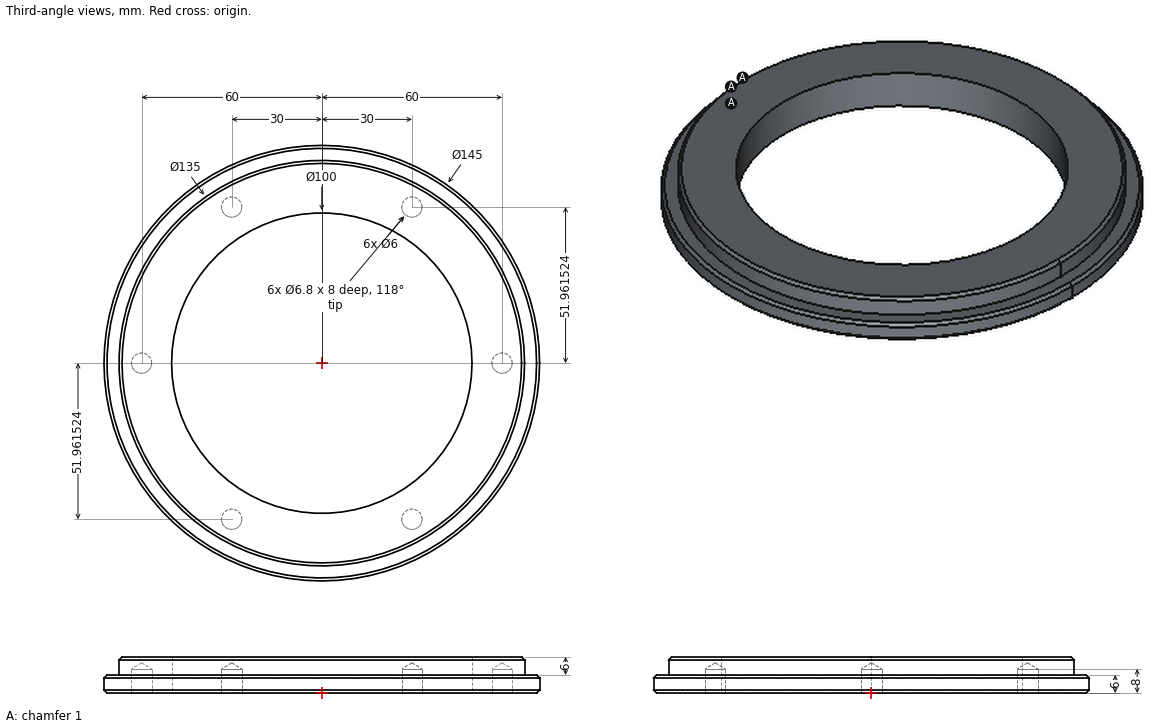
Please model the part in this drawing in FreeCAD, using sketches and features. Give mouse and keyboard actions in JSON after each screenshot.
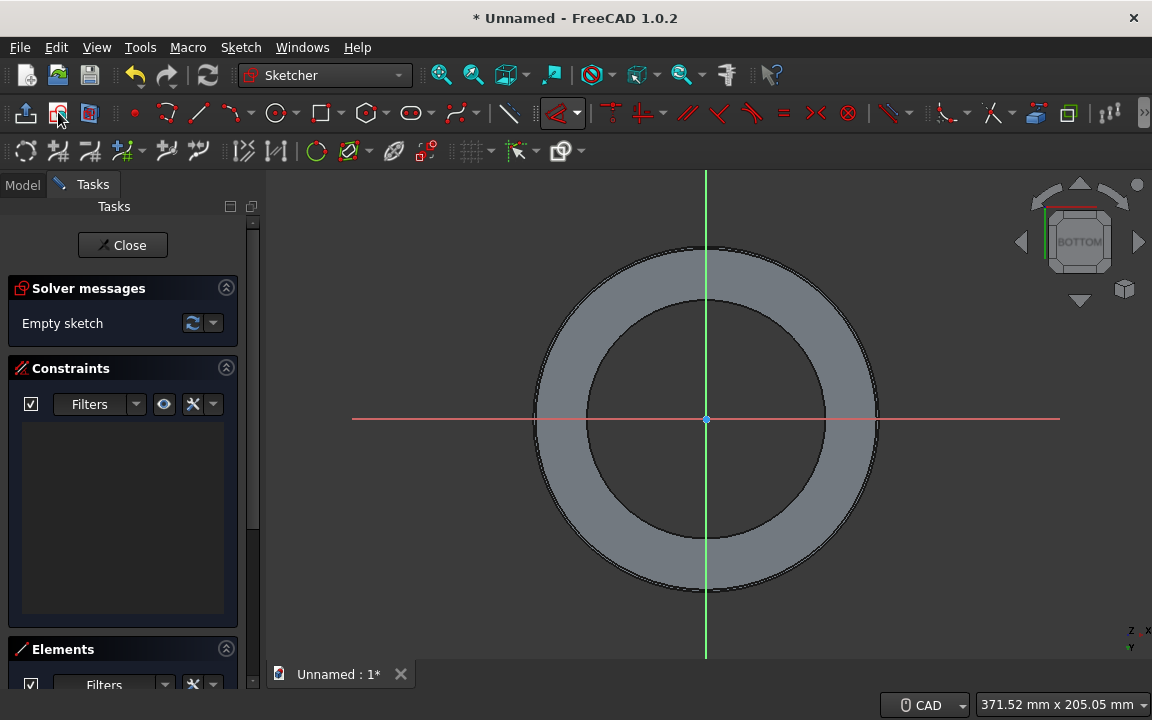
{"action": "left_click", "coordinate": [276, 114]}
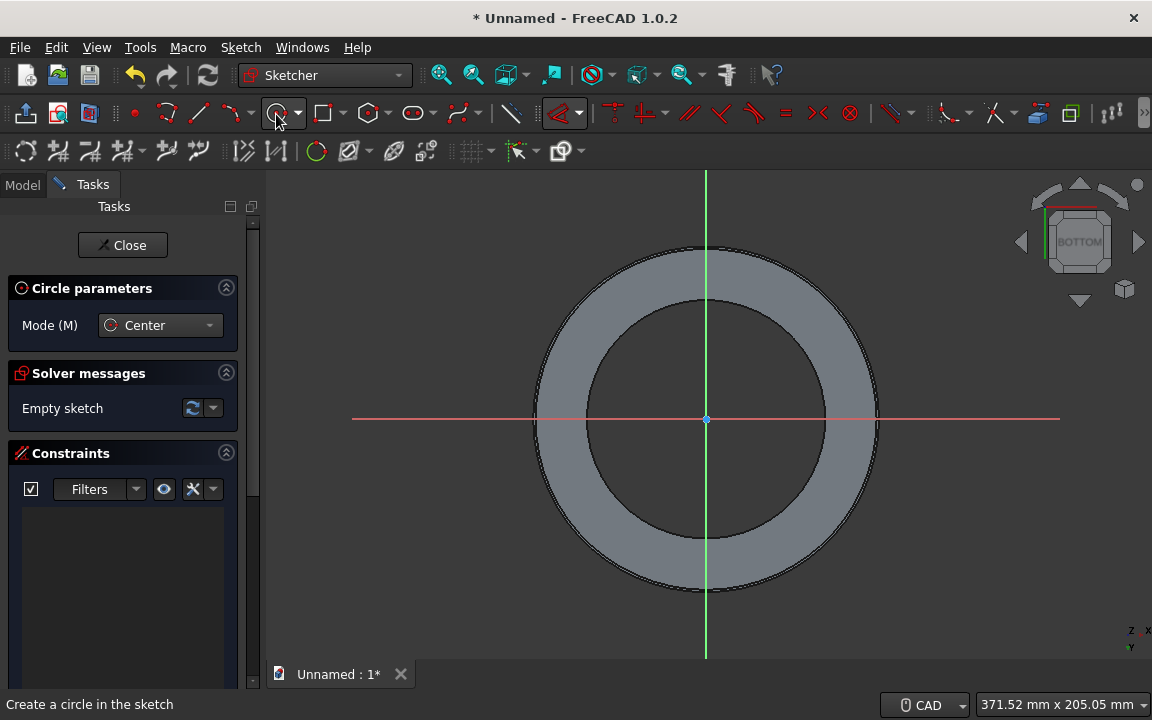
{"action": "scroll", "coordinate": [778, 543], "scroll_direction": "up", "scroll_amount": 6}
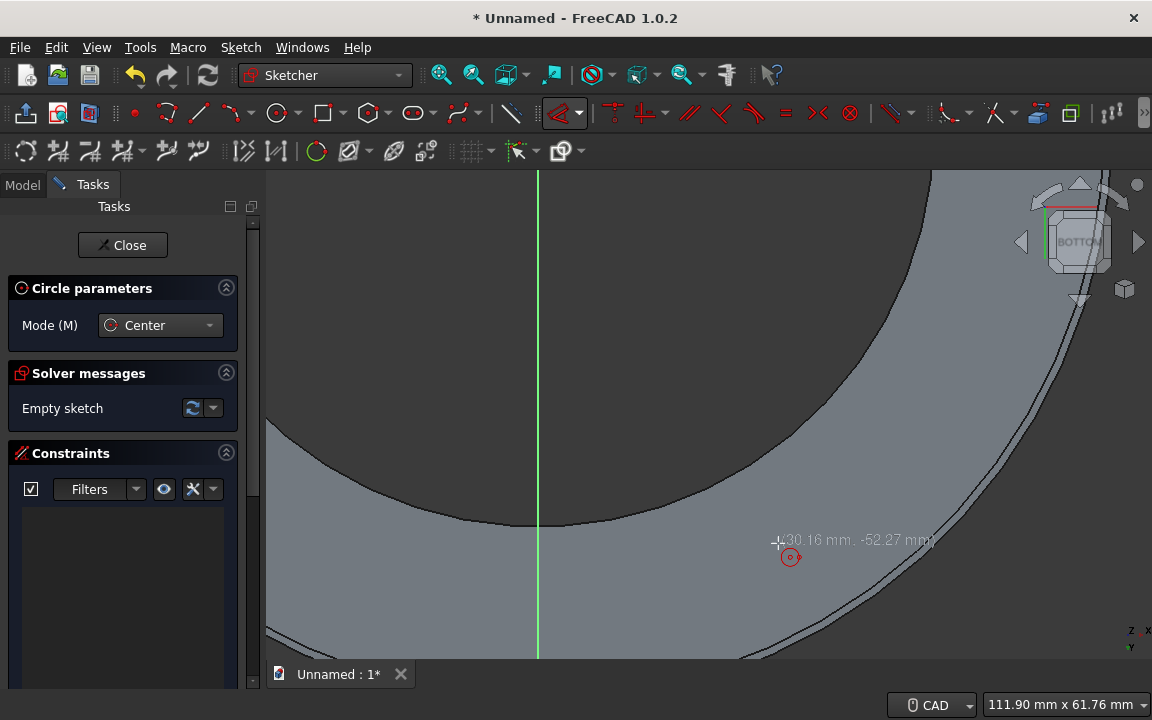
{"action": "left_click", "coordinate": [775, 542]}
{"action": "mouse_move", "coordinate": [792, 525]}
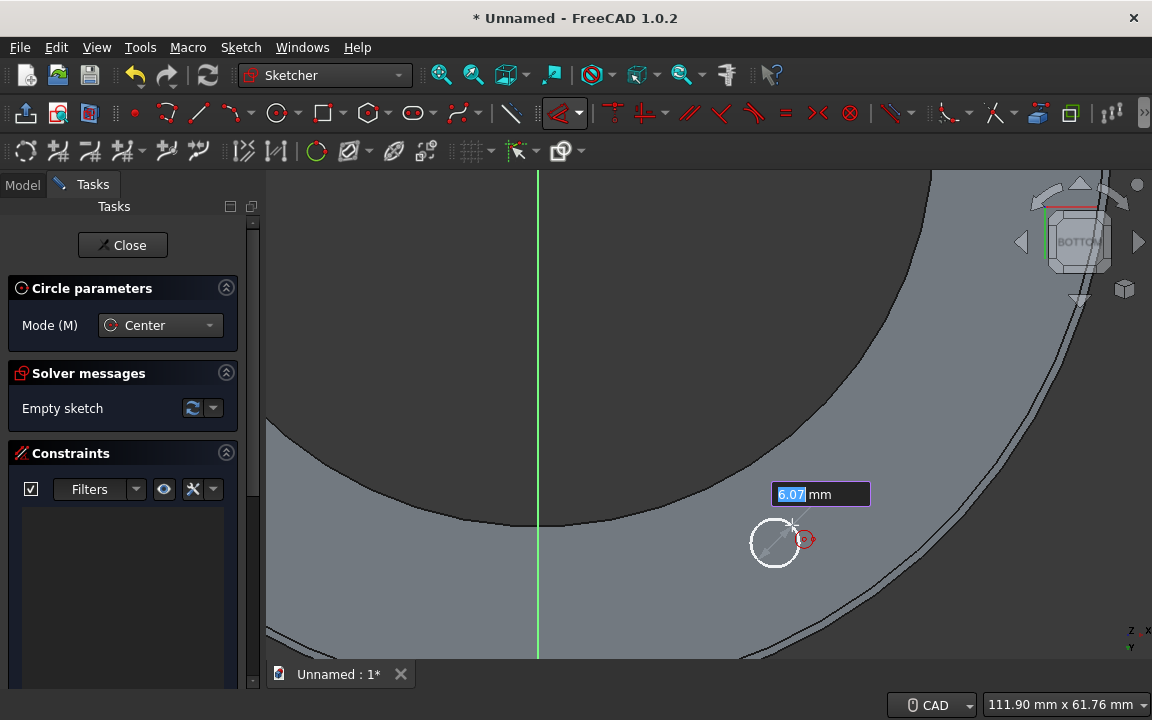
{"action": "type", "text": "6"}
{"action": "key", "text": "Return"}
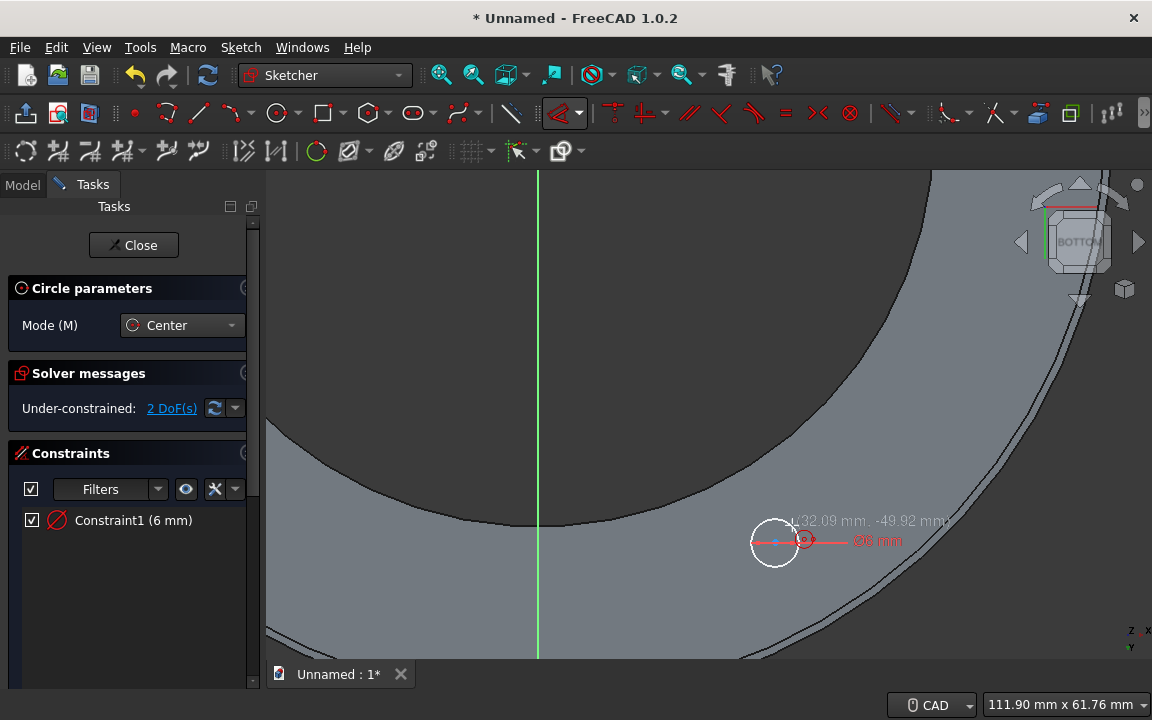
{"action": "scroll", "coordinate": [700, 580], "scroll_direction": "down", "scroll_amount": 5}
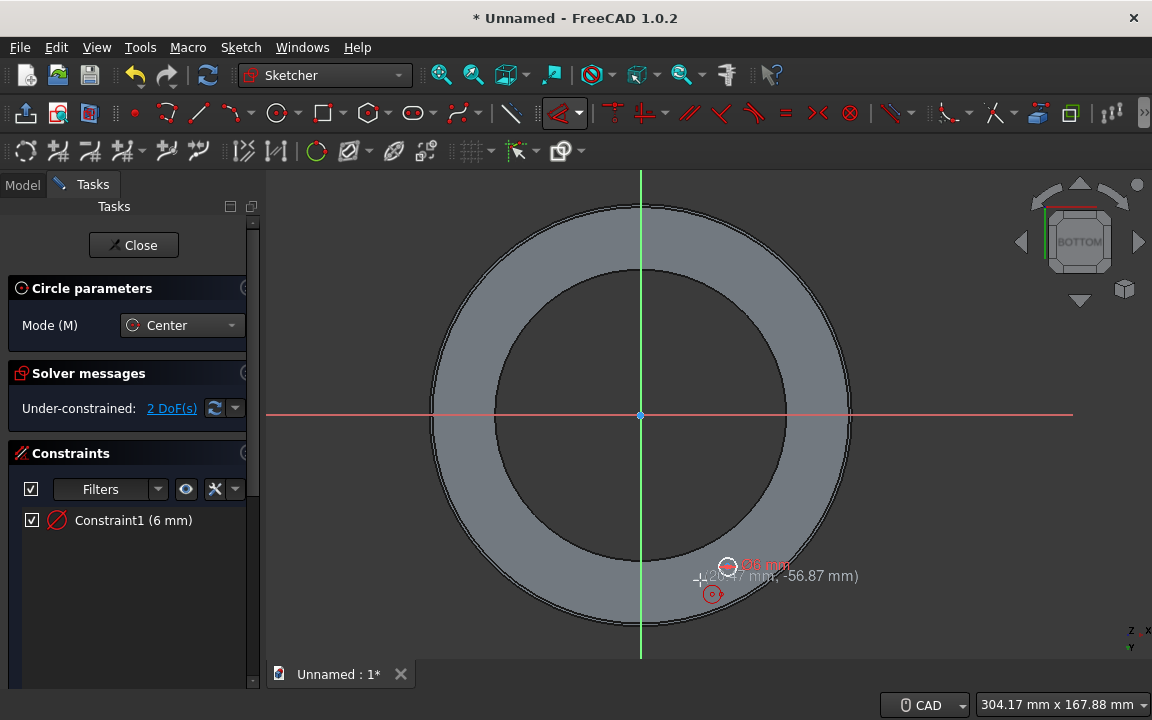
{"action": "scroll", "coordinate": [815, 415], "scroll_direction": "up", "scroll_amount": 5}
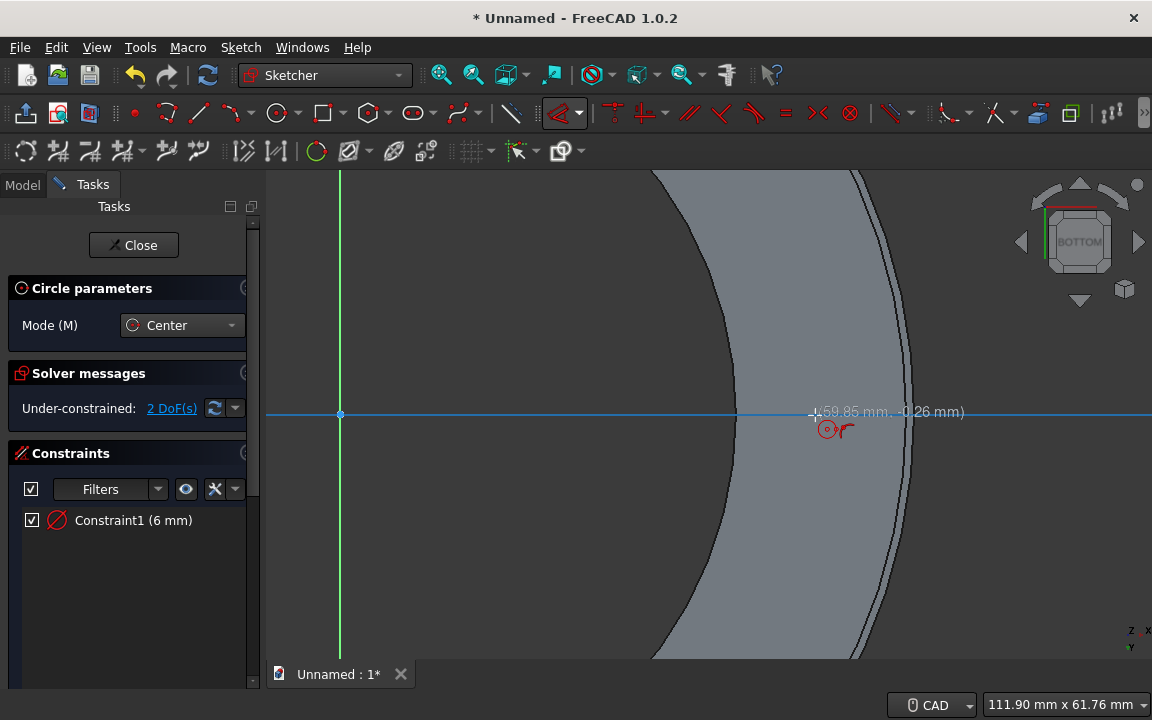
{"action": "left_click", "coordinate": [815, 415]}
{"action": "mouse_move", "coordinate": [832, 398]}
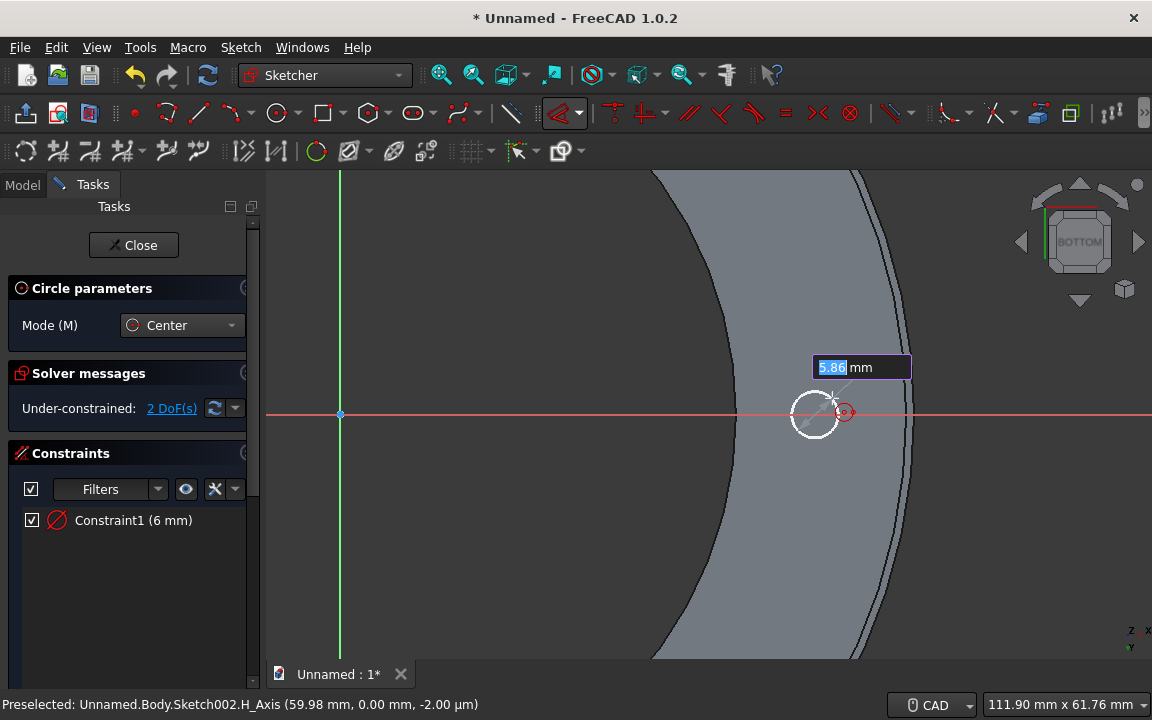
{"action": "type", "text": "6"}
{"action": "key", "text": "Return"}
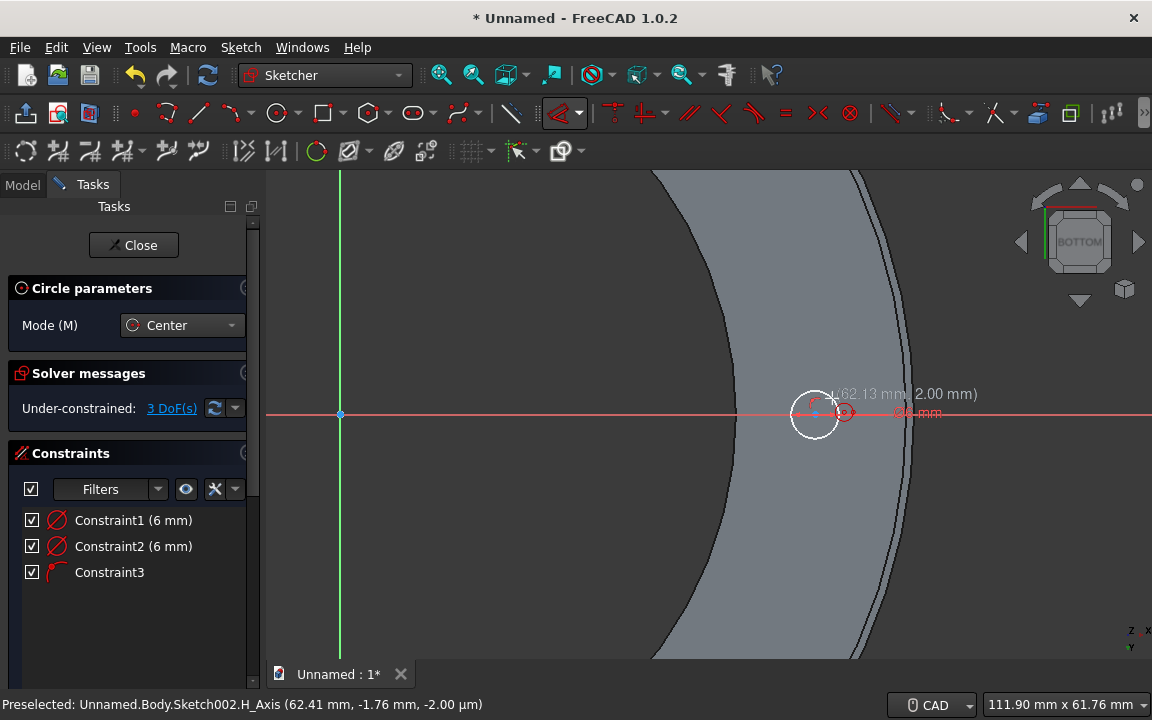
{"action": "scroll", "coordinate": [815, 414], "scroll_direction": "down", "scroll_amount": 5}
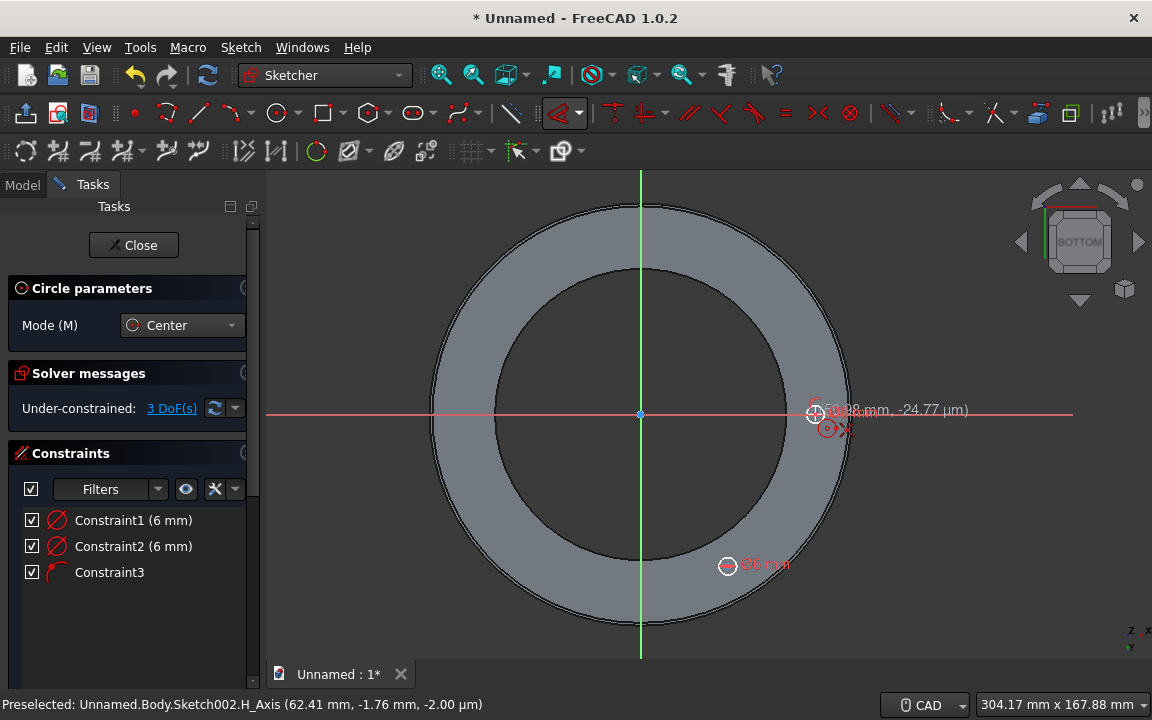
{"action": "scroll", "coordinate": [553, 566], "scroll_direction": "up", "scroll_amount": 5}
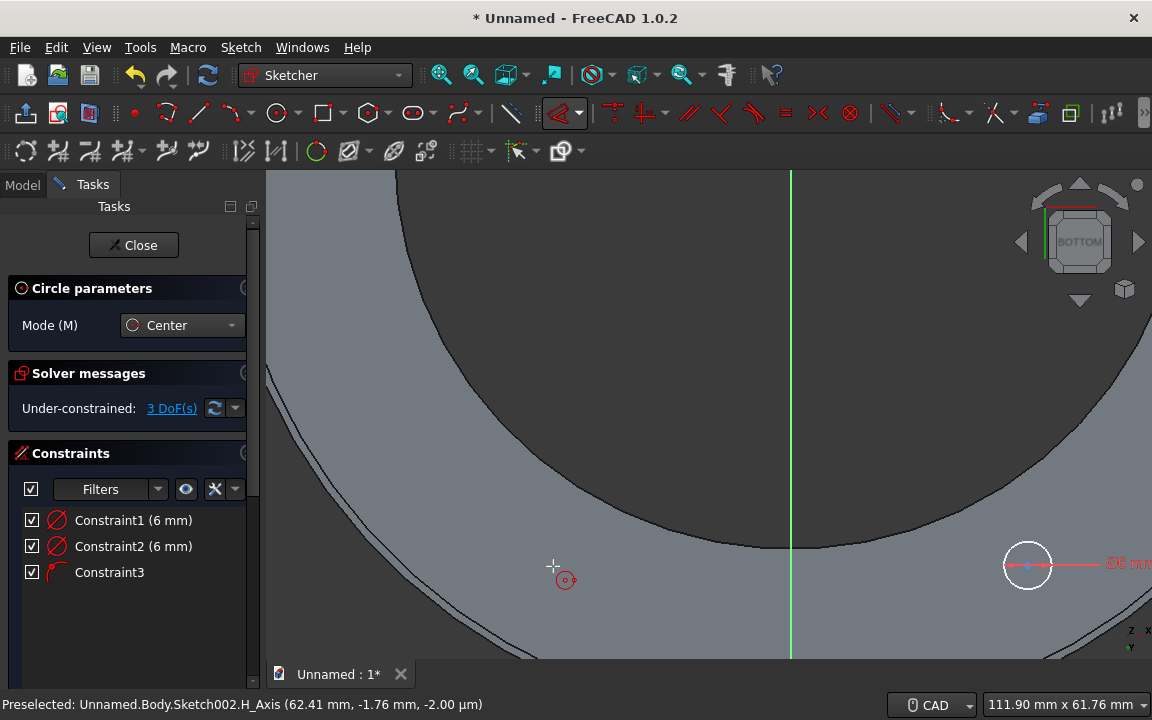
{"action": "left_click", "coordinate": [553, 565]}
{"action": "mouse_move", "coordinate": [570, 548]}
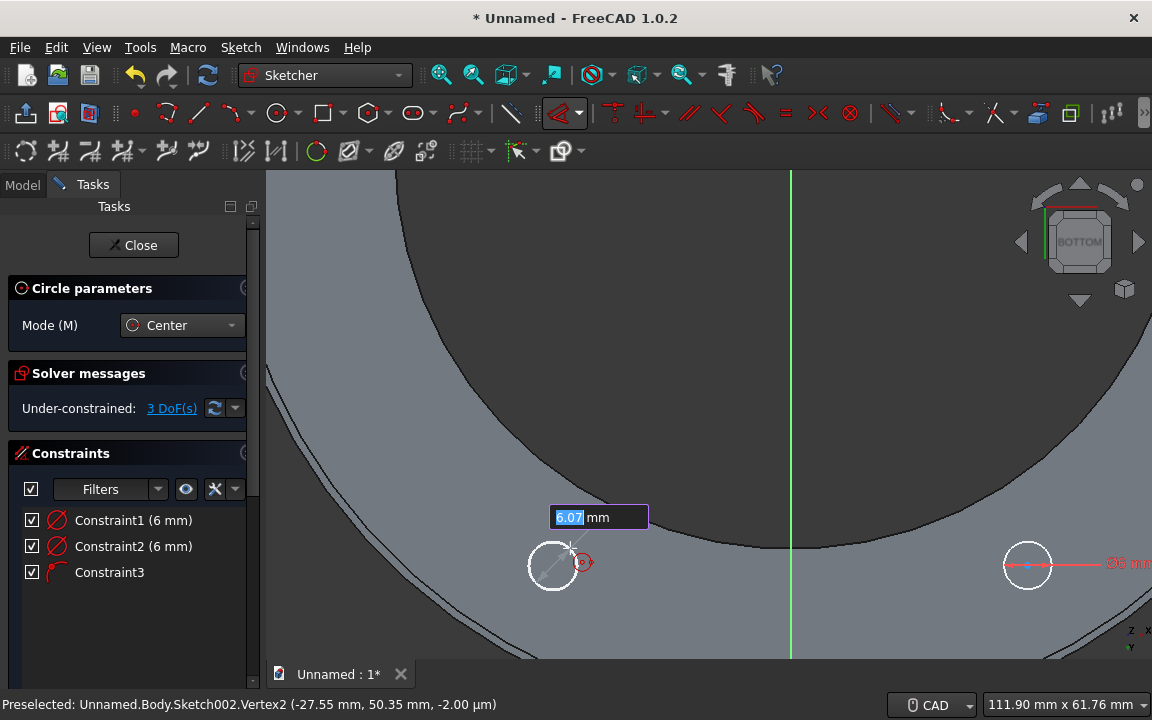
{"action": "type", "text": "6"}
{"action": "key", "text": "Return"}